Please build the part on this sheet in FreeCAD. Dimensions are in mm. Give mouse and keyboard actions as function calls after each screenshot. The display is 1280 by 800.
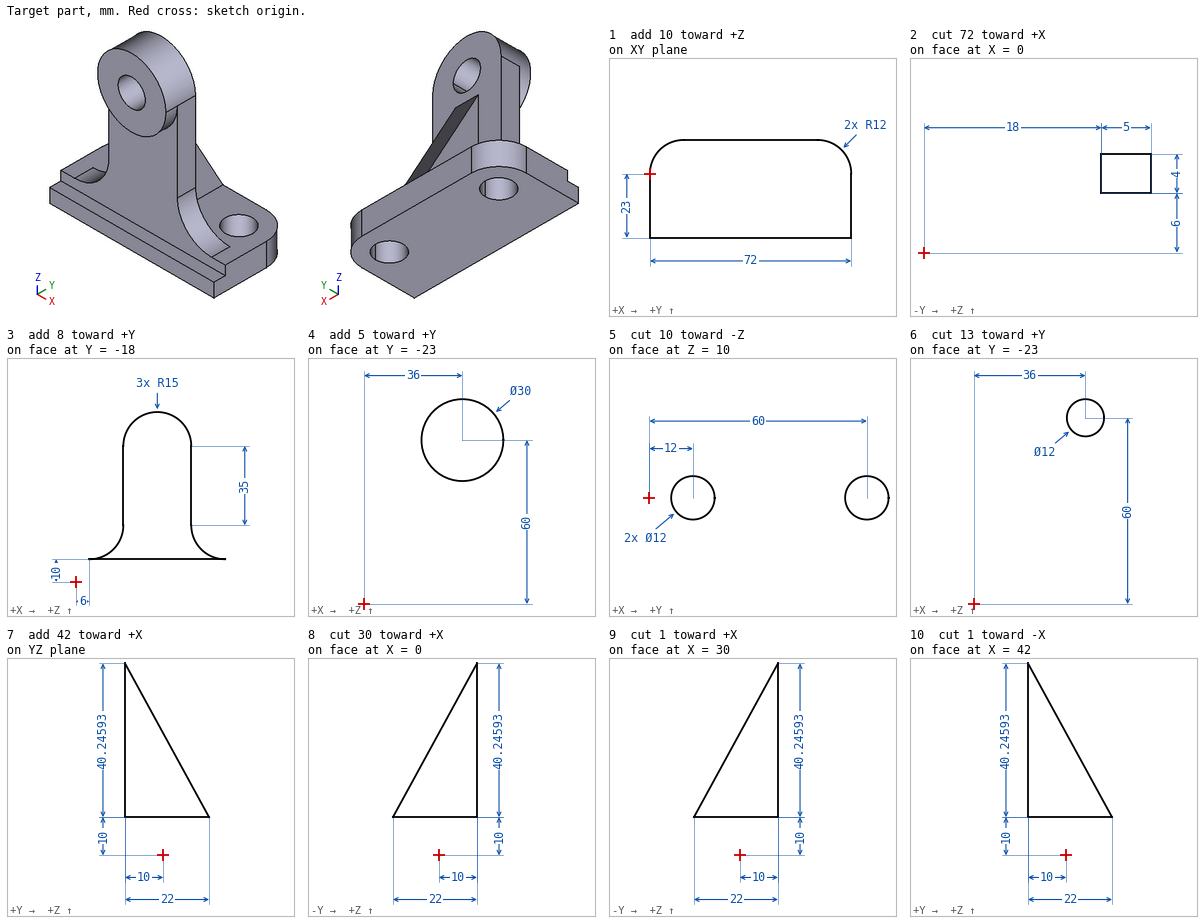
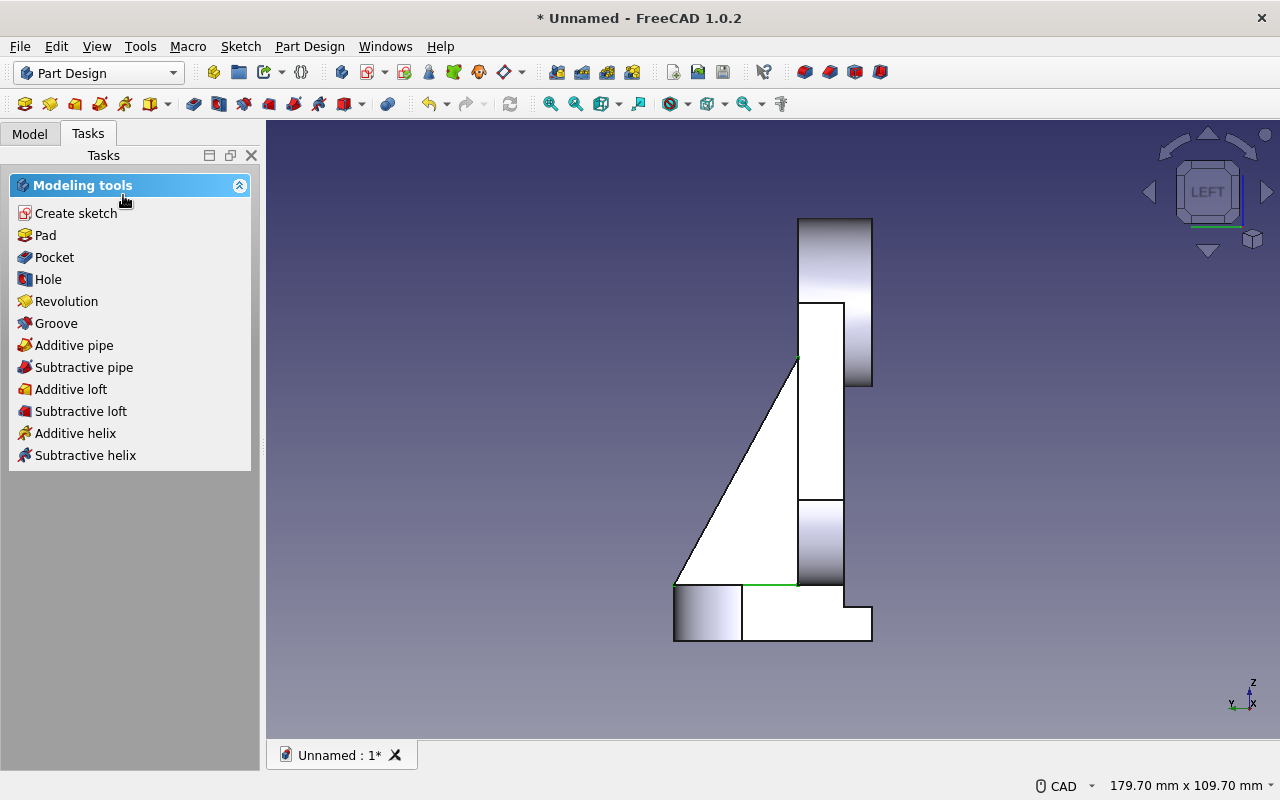
click(194, 104)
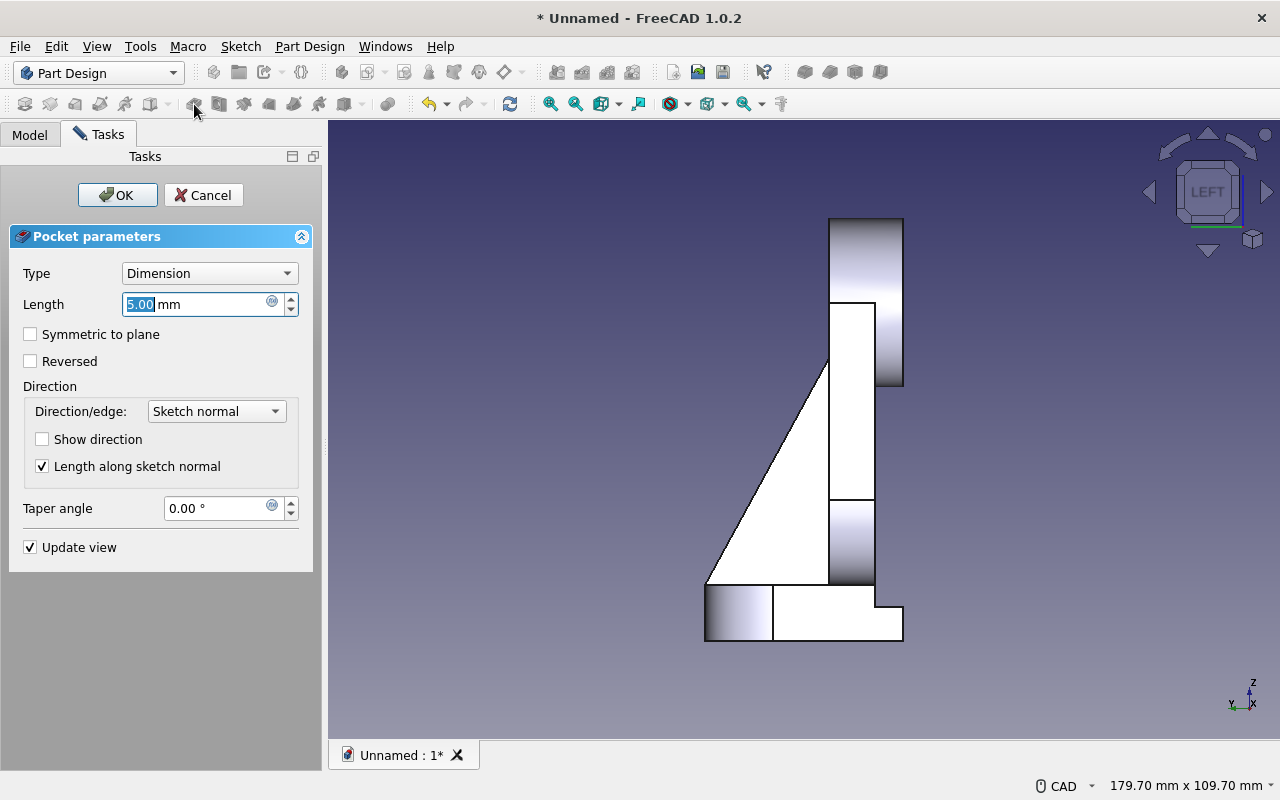
text(30)
key(Tab)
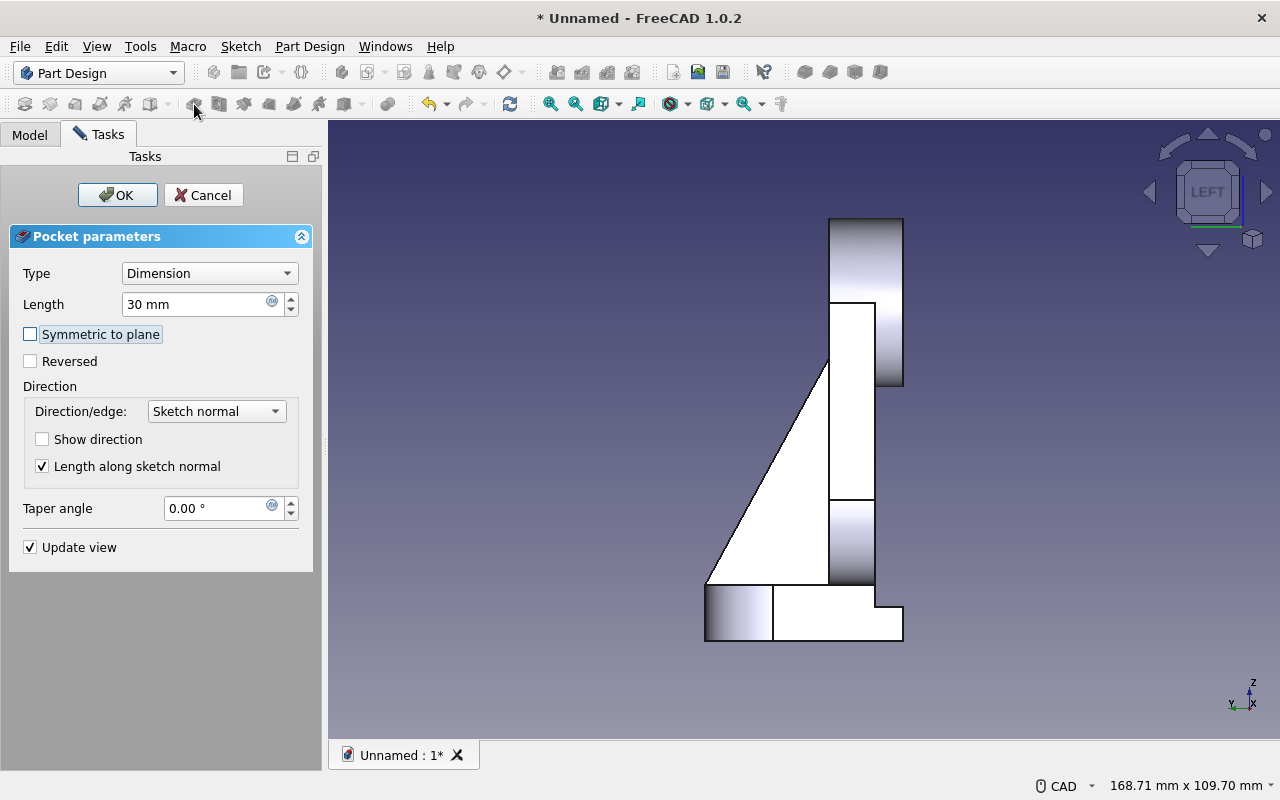
click(118, 195)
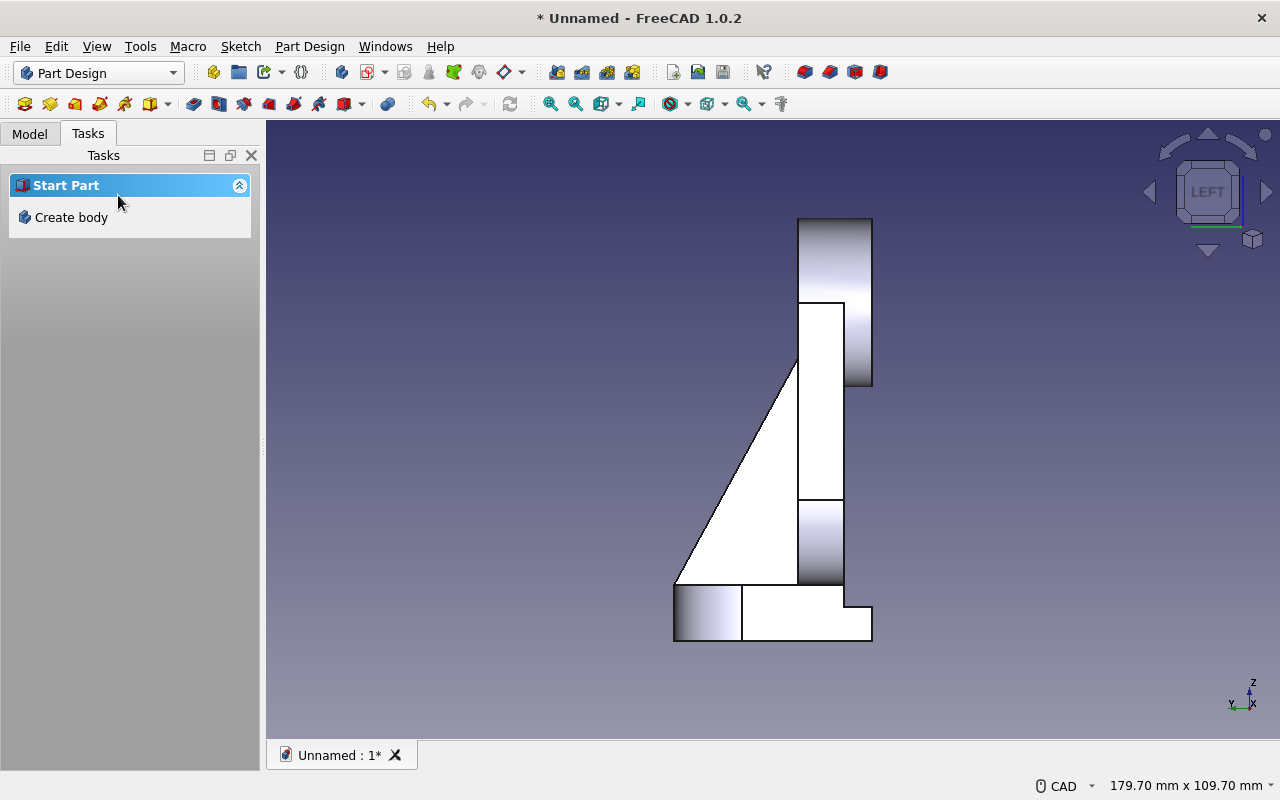
click(754, 535)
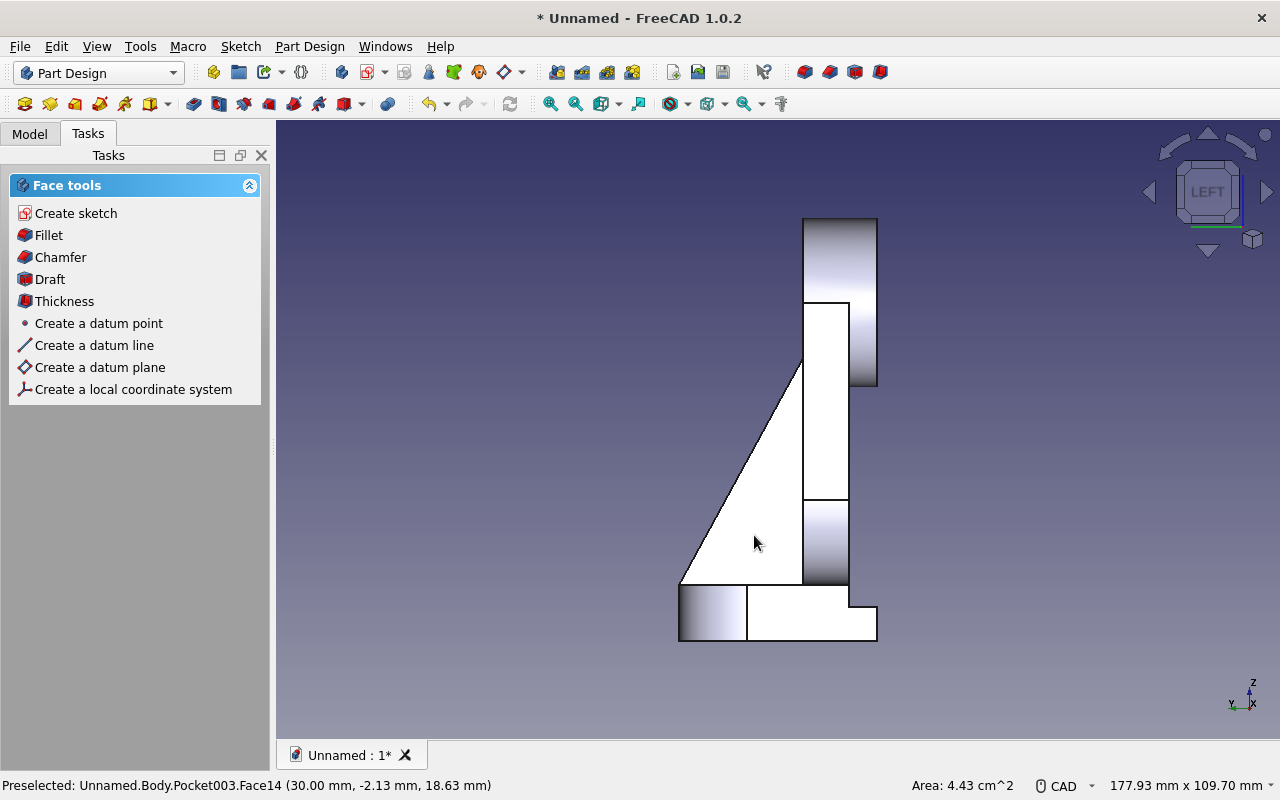
click(366, 72)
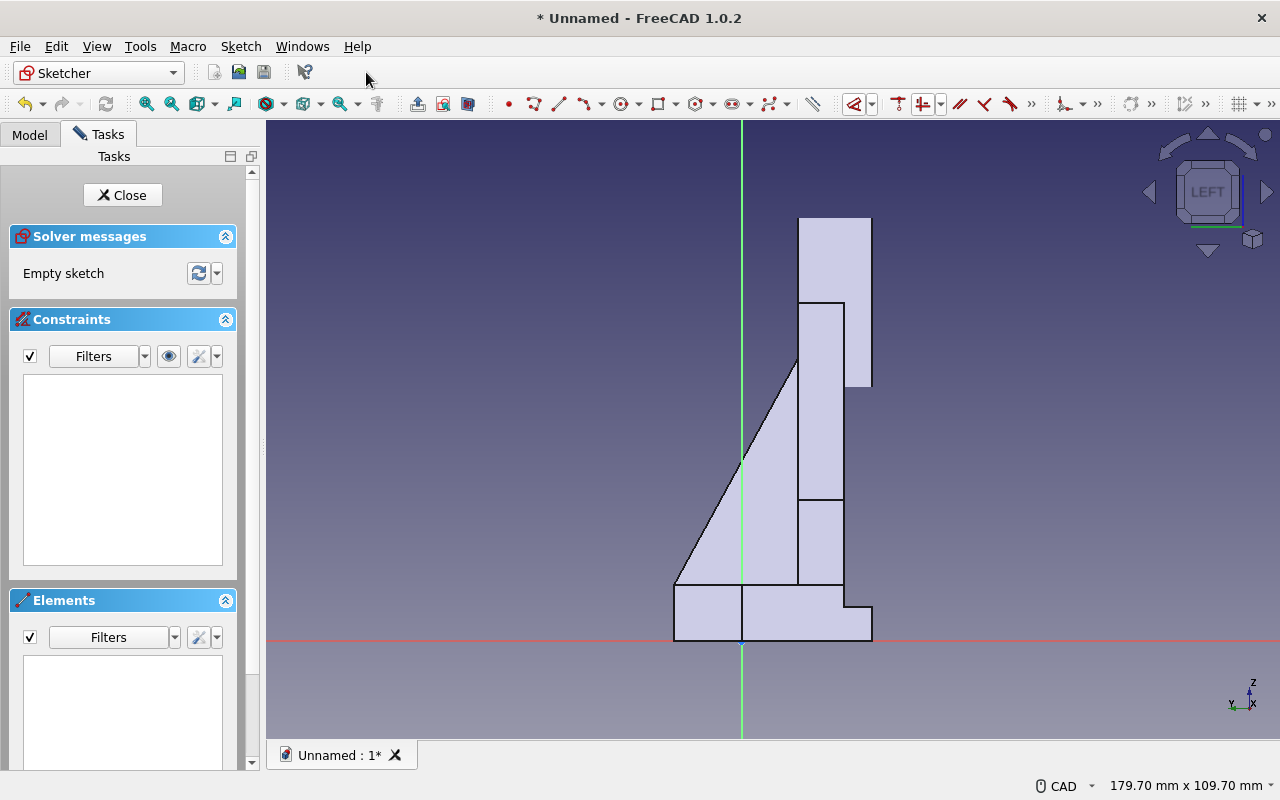
click(468, 104)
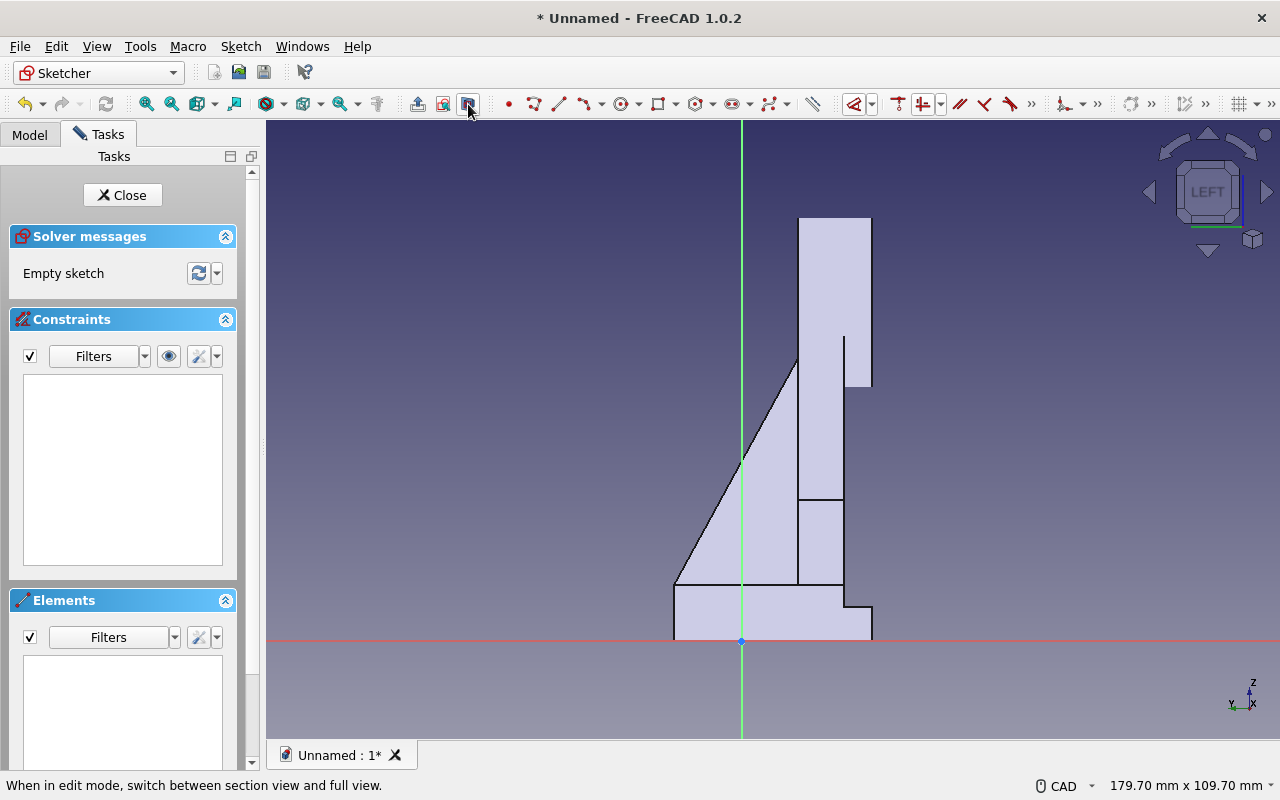
scroll(801, 641, up, 2)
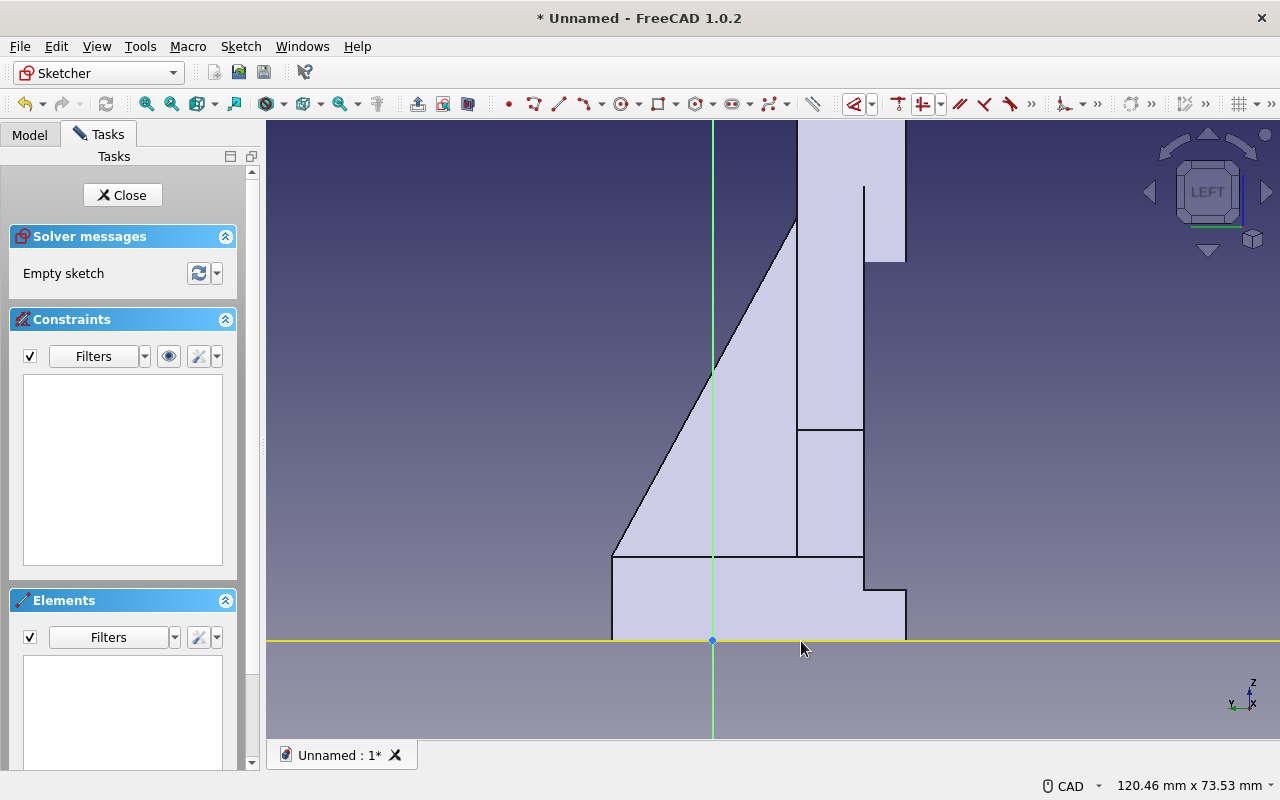
click(534, 104)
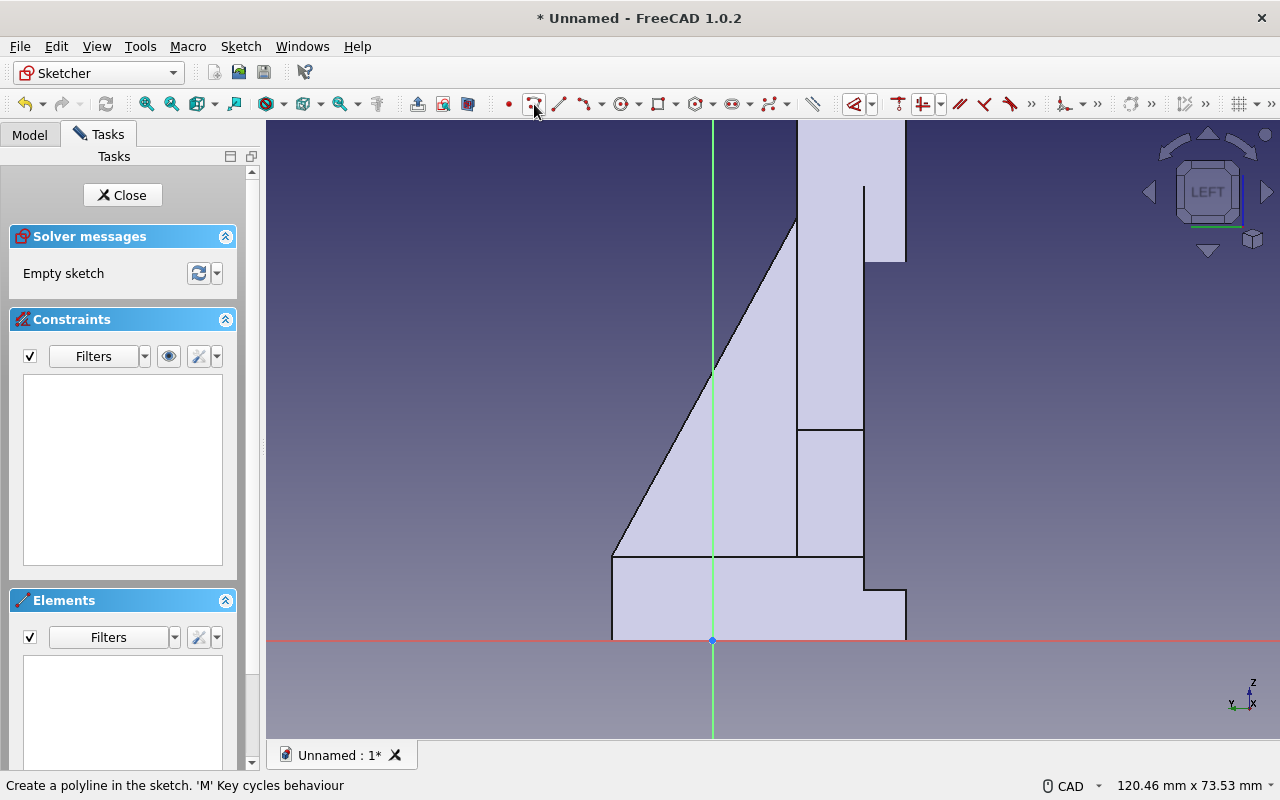
click(797, 557)
click(797, 218)
click(612, 557)
click(797, 558)
key(Escape)
key(Escape)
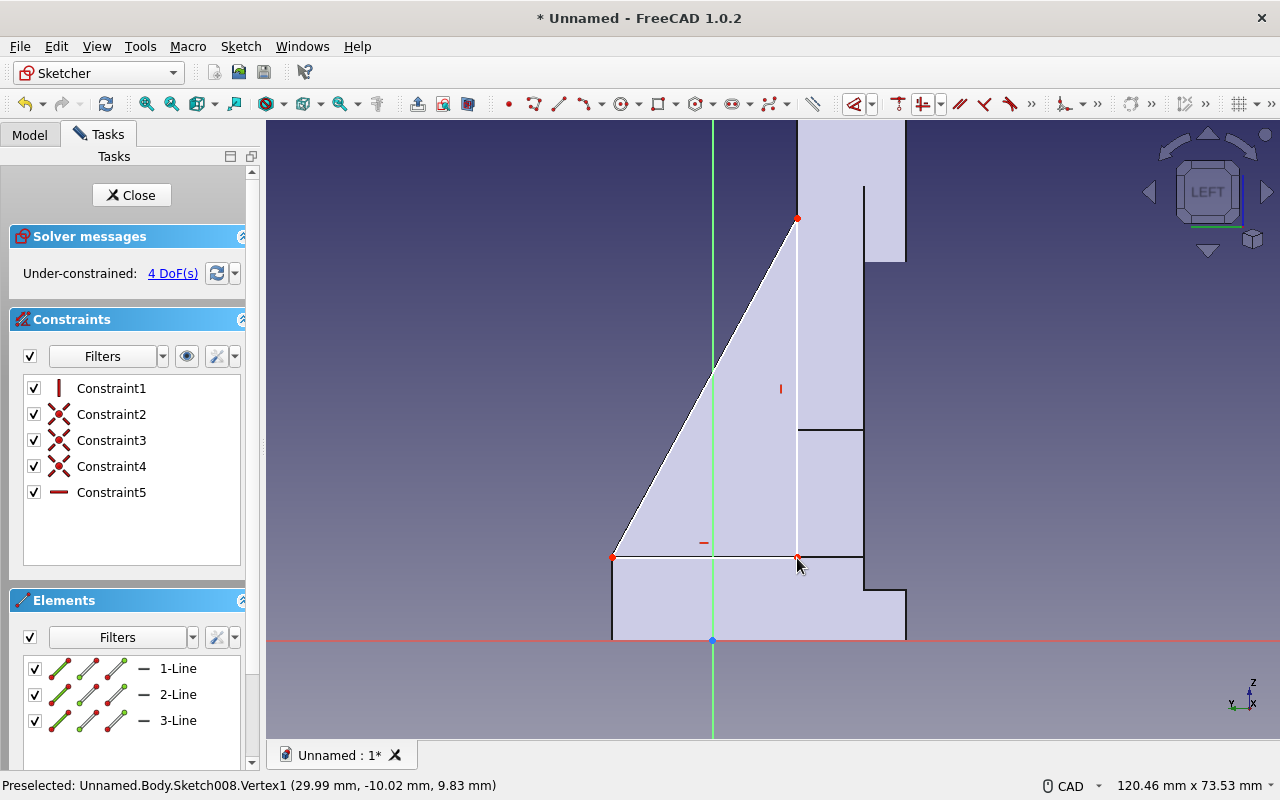
click(667, 558)